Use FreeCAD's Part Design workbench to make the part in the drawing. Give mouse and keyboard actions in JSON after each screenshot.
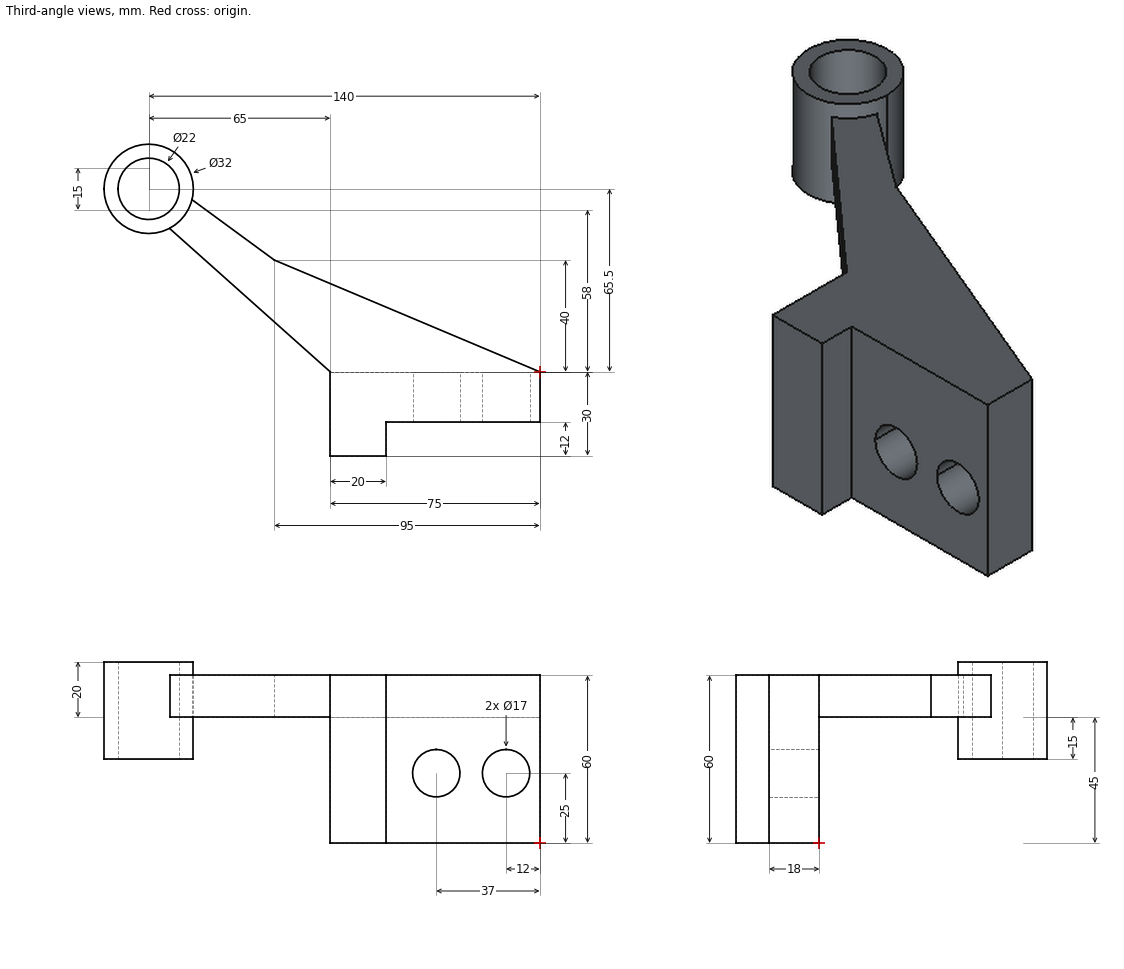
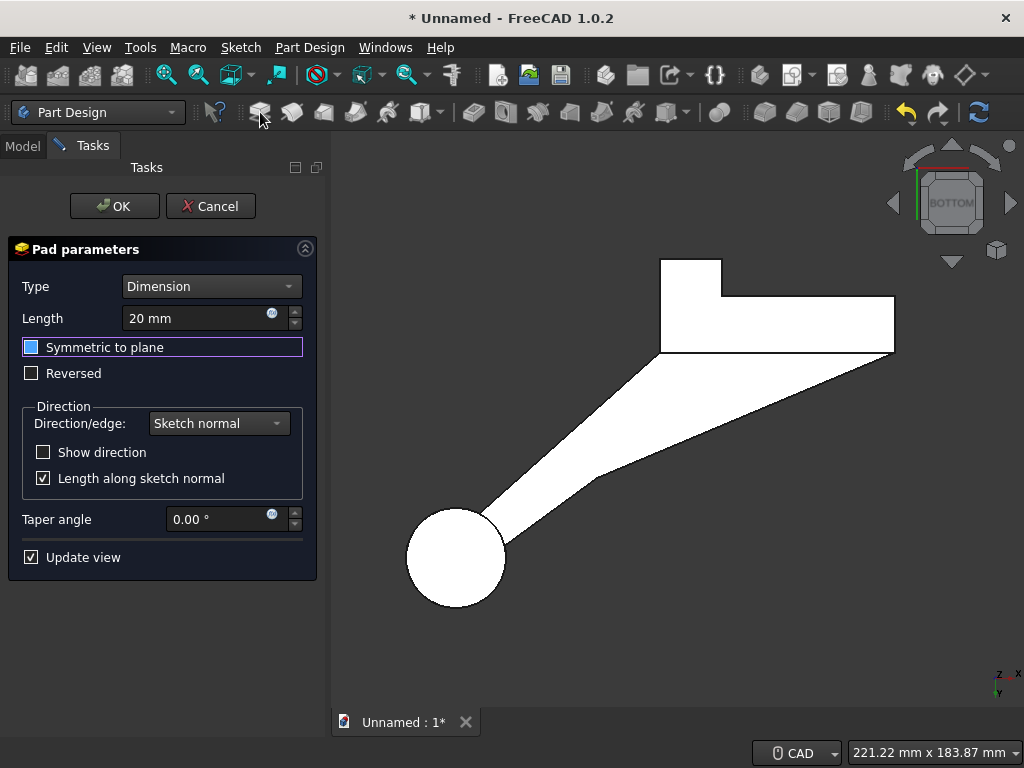
{"action": "left_click", "coordinate": [30, 373]}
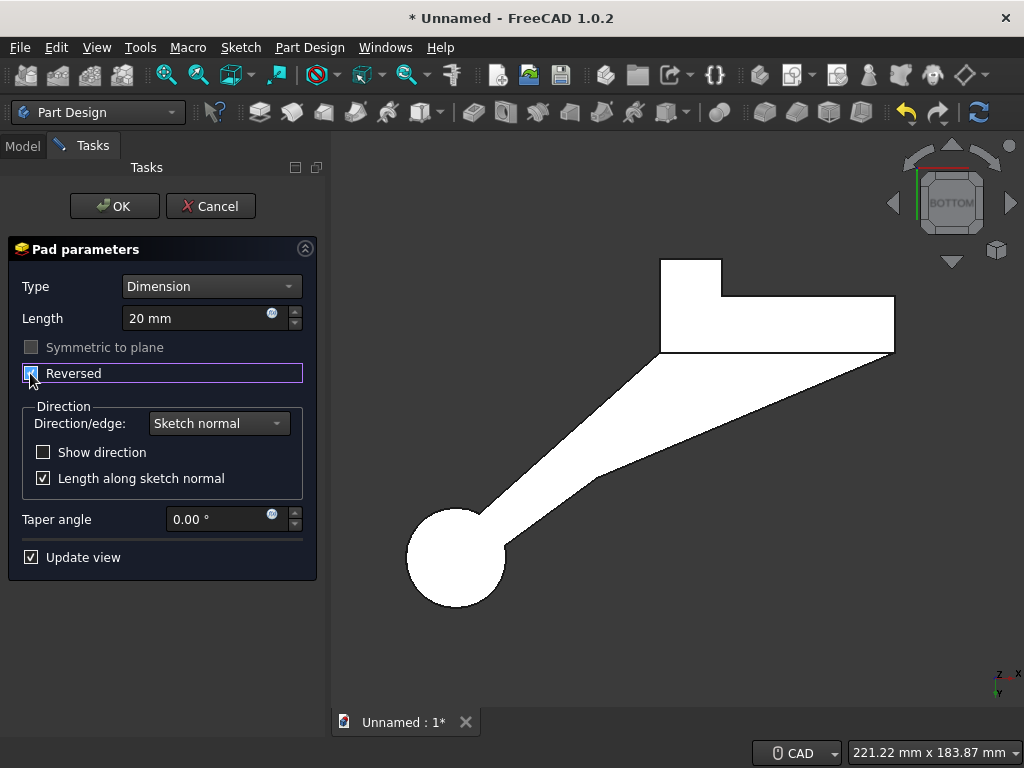
{"action": "left_click", "coordinate": [115, 206]}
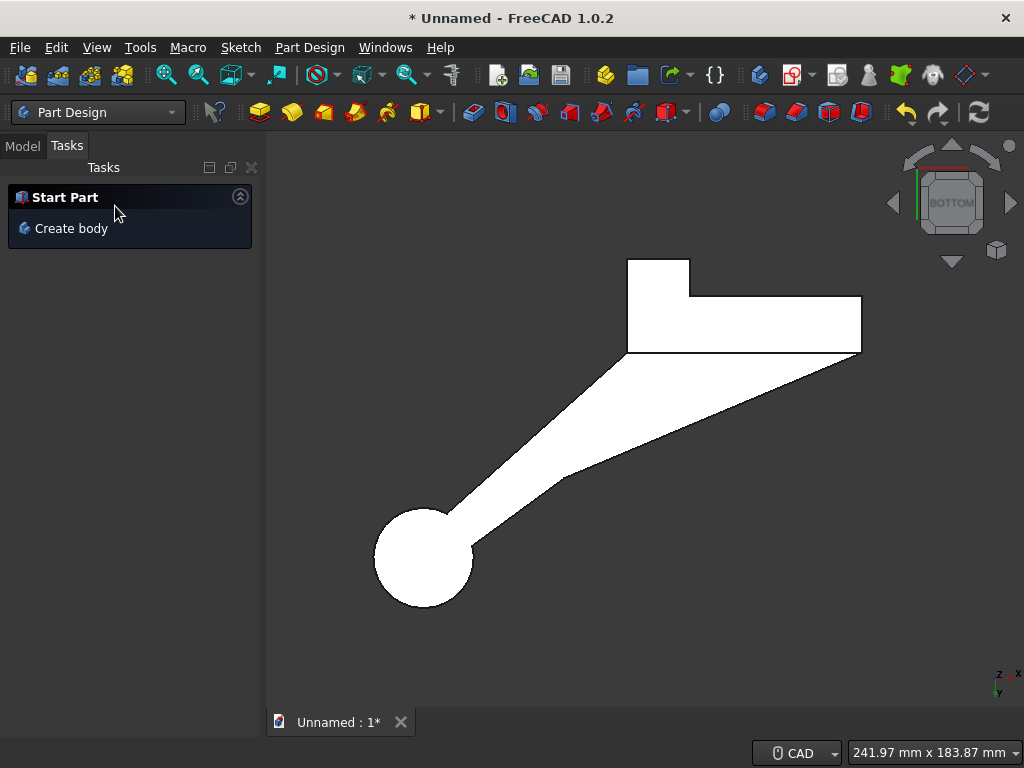
{"action": "left_click", "coordinate": [23, 145]}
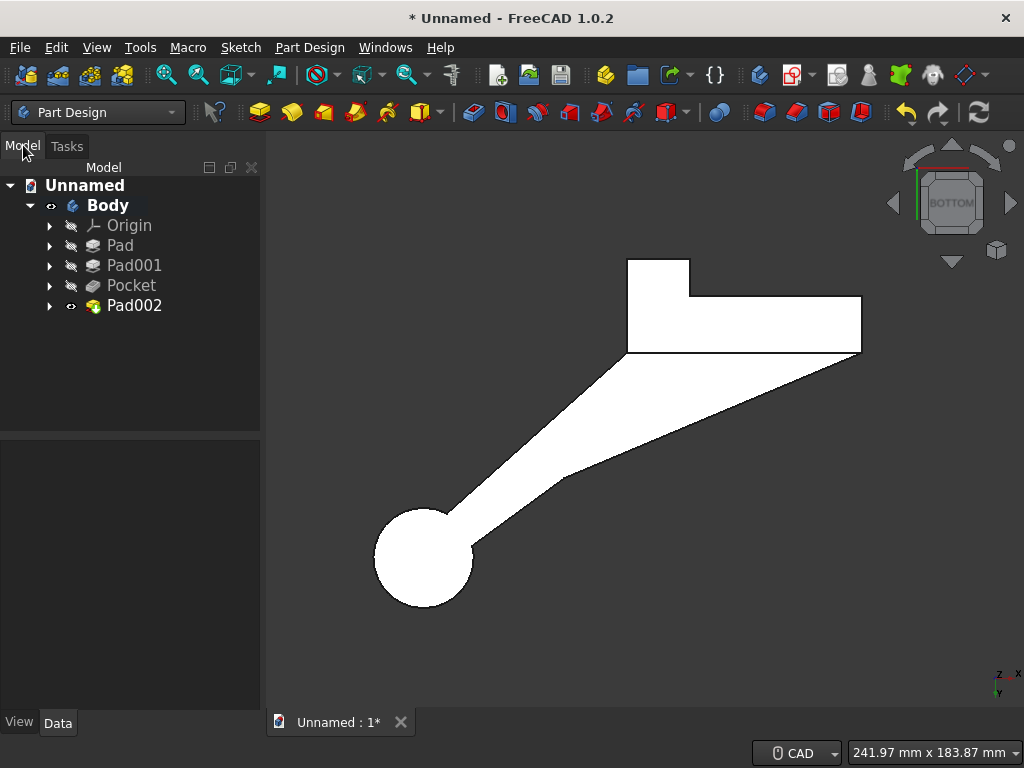
{"action": "left_click", "coordinate": [50, 226]}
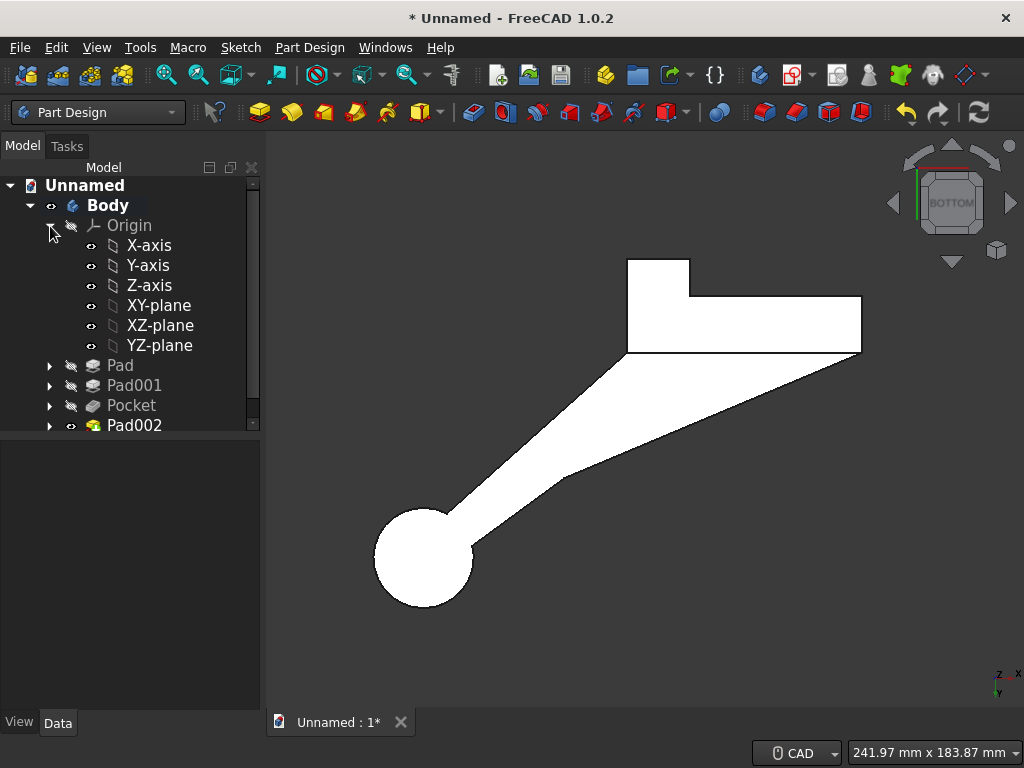
{"action": "left_click", "coordinate": [136, 306]}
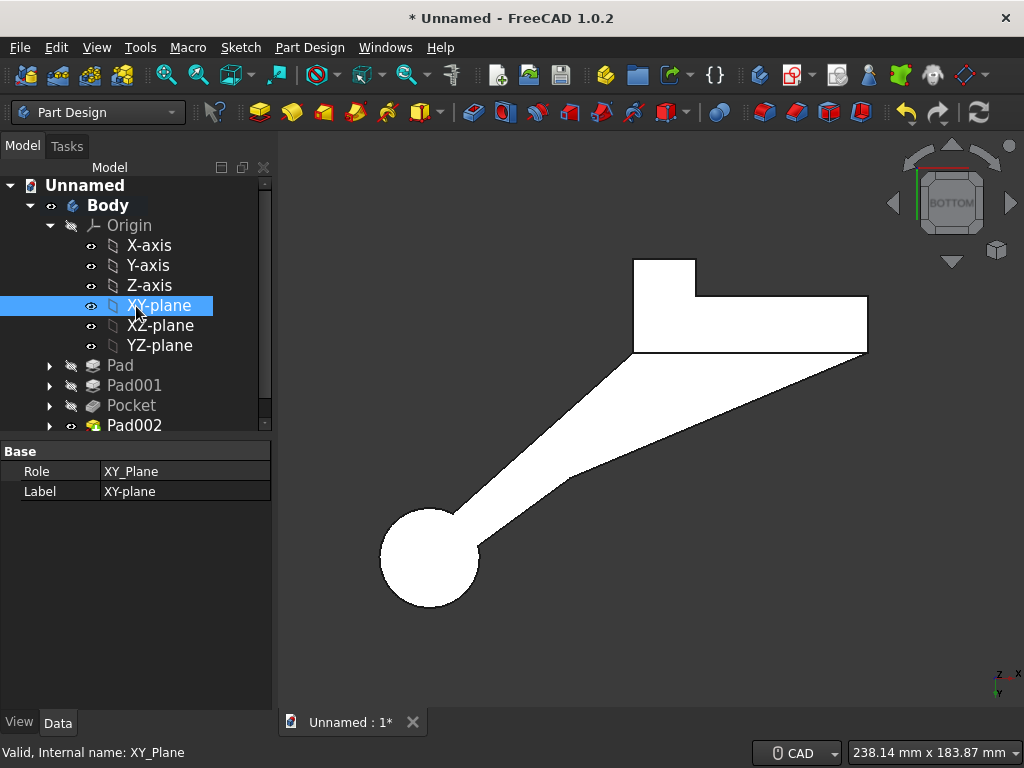
{"action": "left_click", "coordinate": [966, 76]}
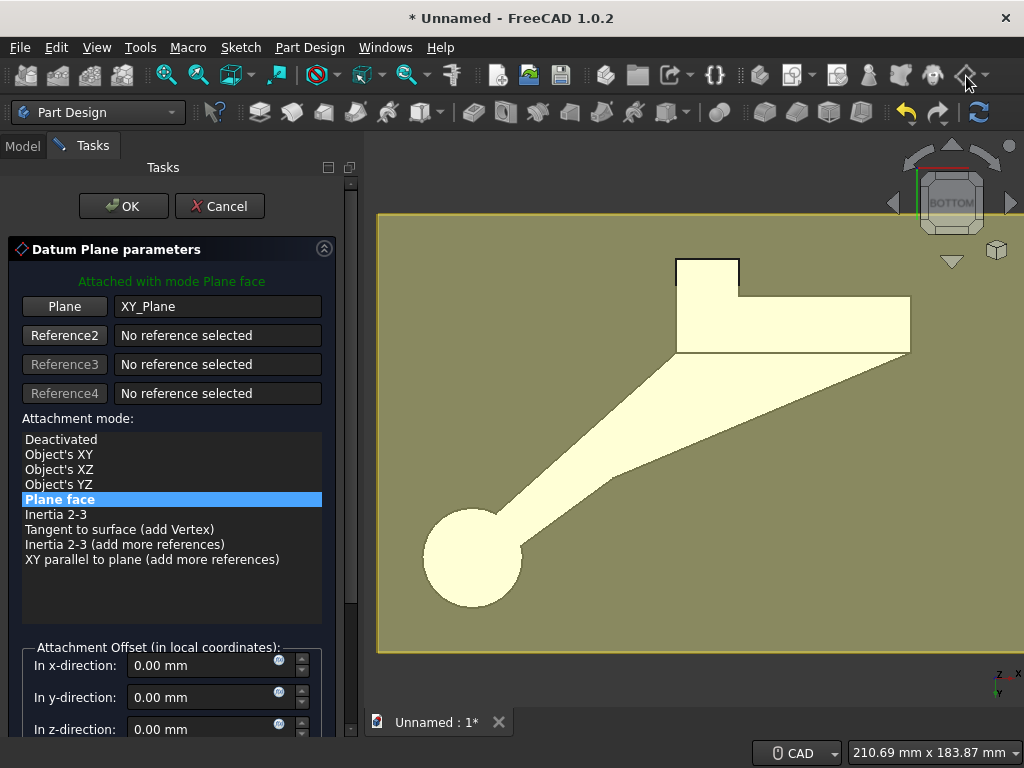
{"action": "scroll", "coordinate": [351, 456], "scroll_direction": "down", "scroll_amount": 2}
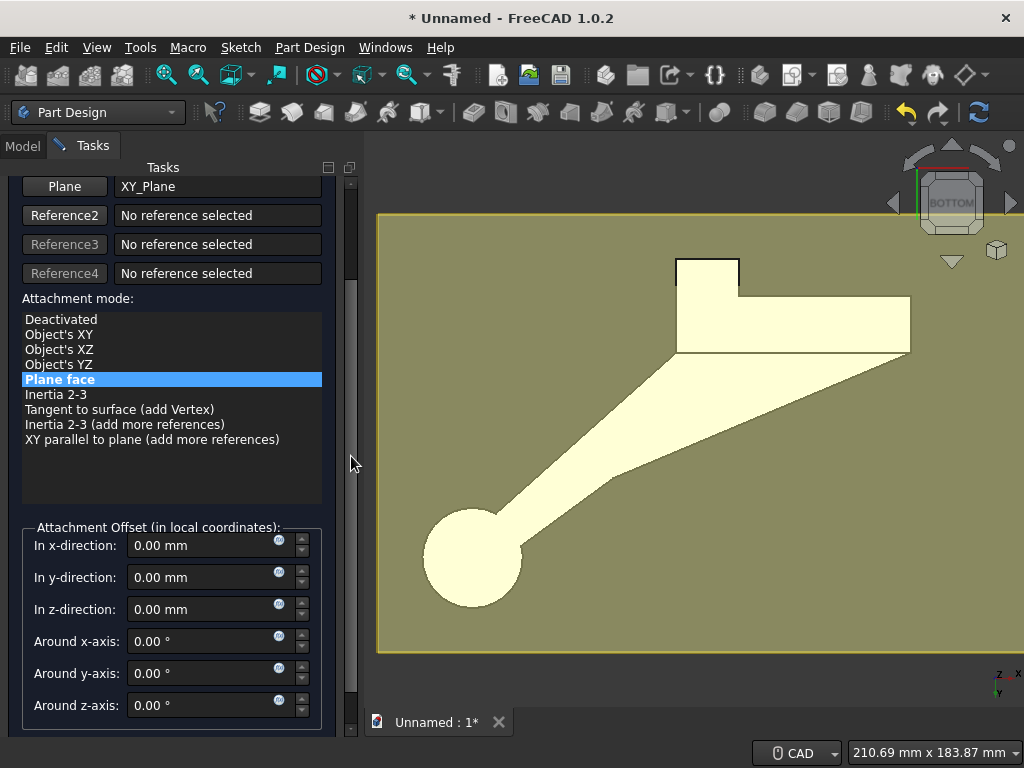
{"action": "triple_click", "coordinate": [210, 609]}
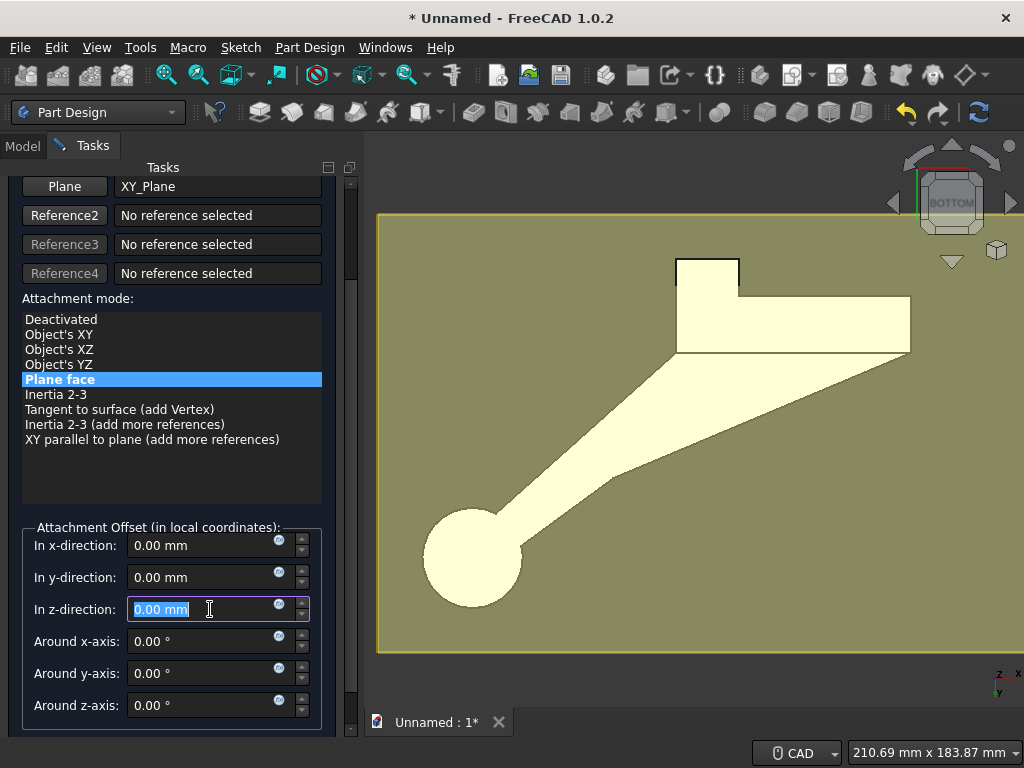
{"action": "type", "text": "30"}
{"action": "key", "text": "Tab"}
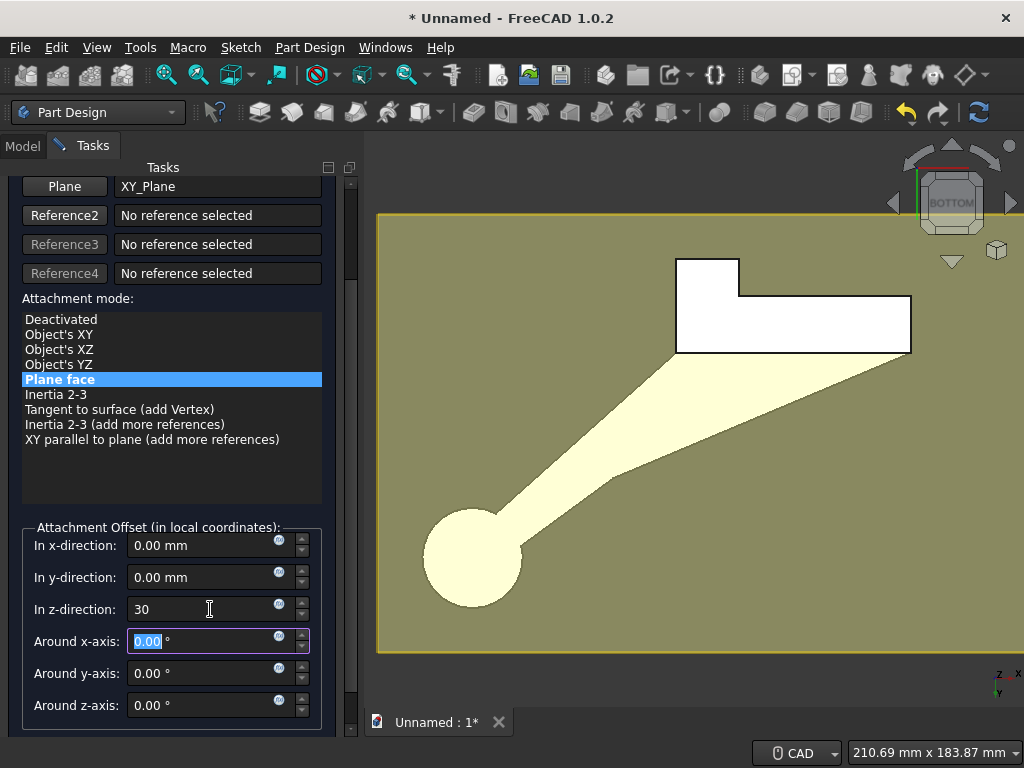
{"action": "scroll", "coordinate": [351, 456], "scroll_direction": "up", "scroll_amount": 3}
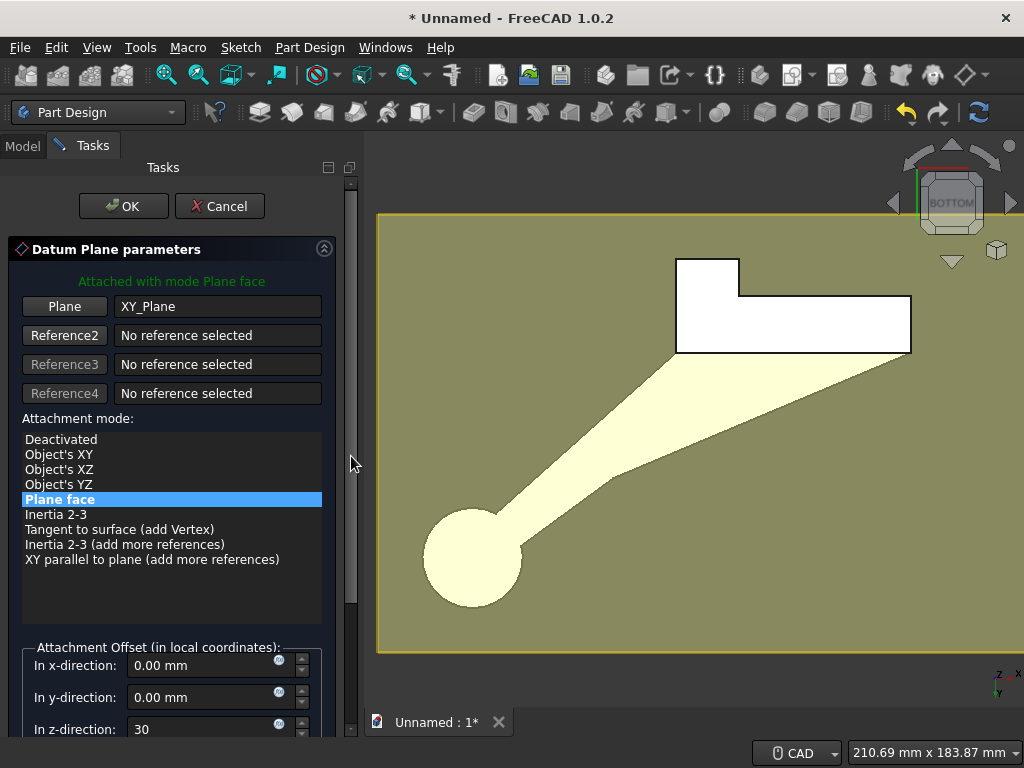
{"action": "left_click", "coordinate": [124, 206]}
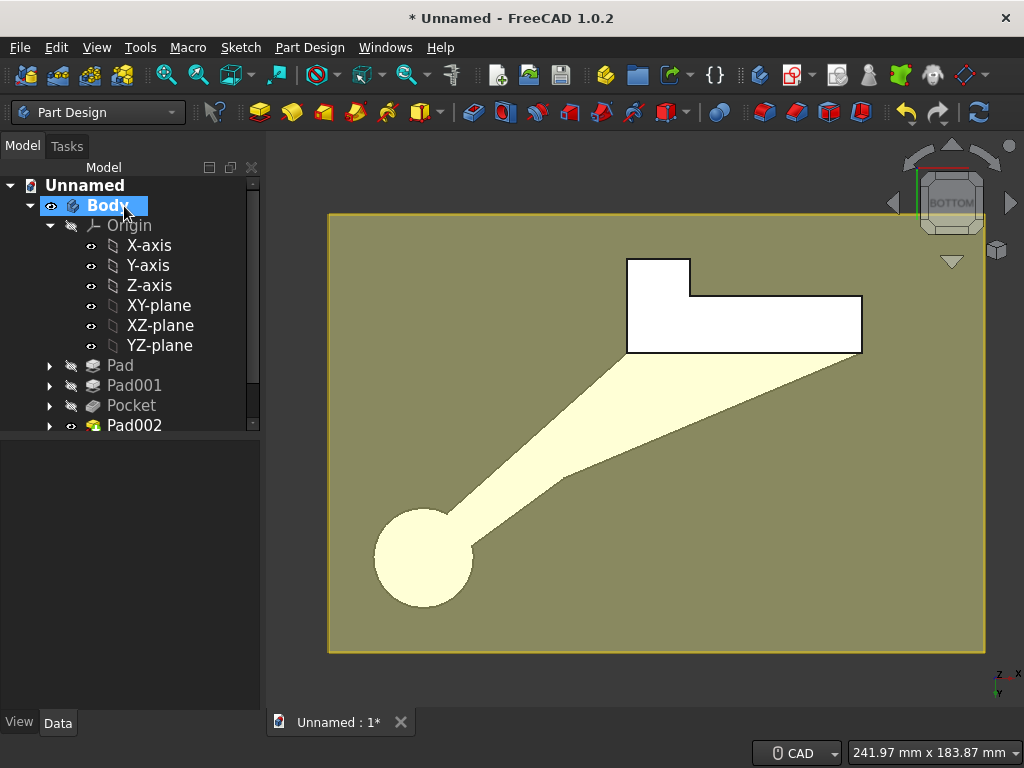
{"action": "scroll", "coordinate": [100, 301], "scroll_direction": "down", "scroll_amount": 3}